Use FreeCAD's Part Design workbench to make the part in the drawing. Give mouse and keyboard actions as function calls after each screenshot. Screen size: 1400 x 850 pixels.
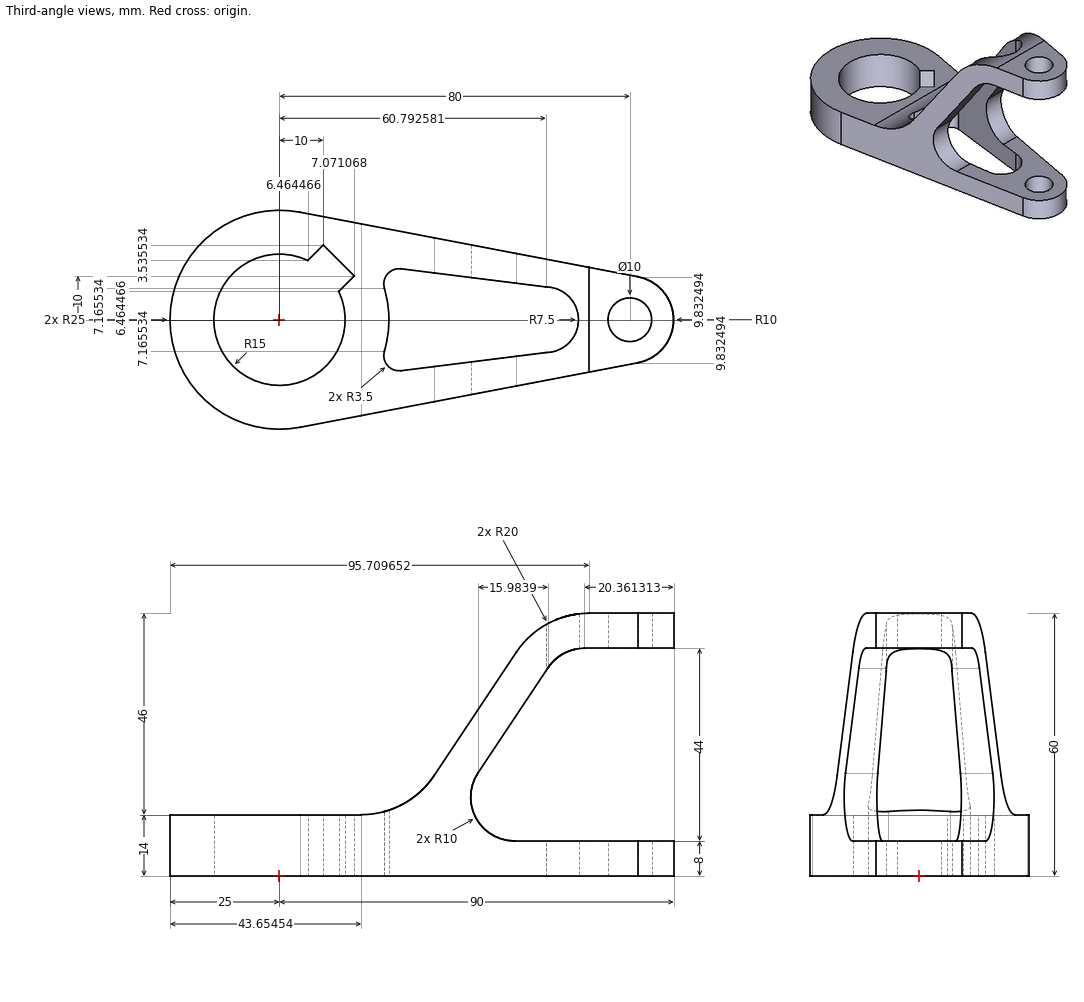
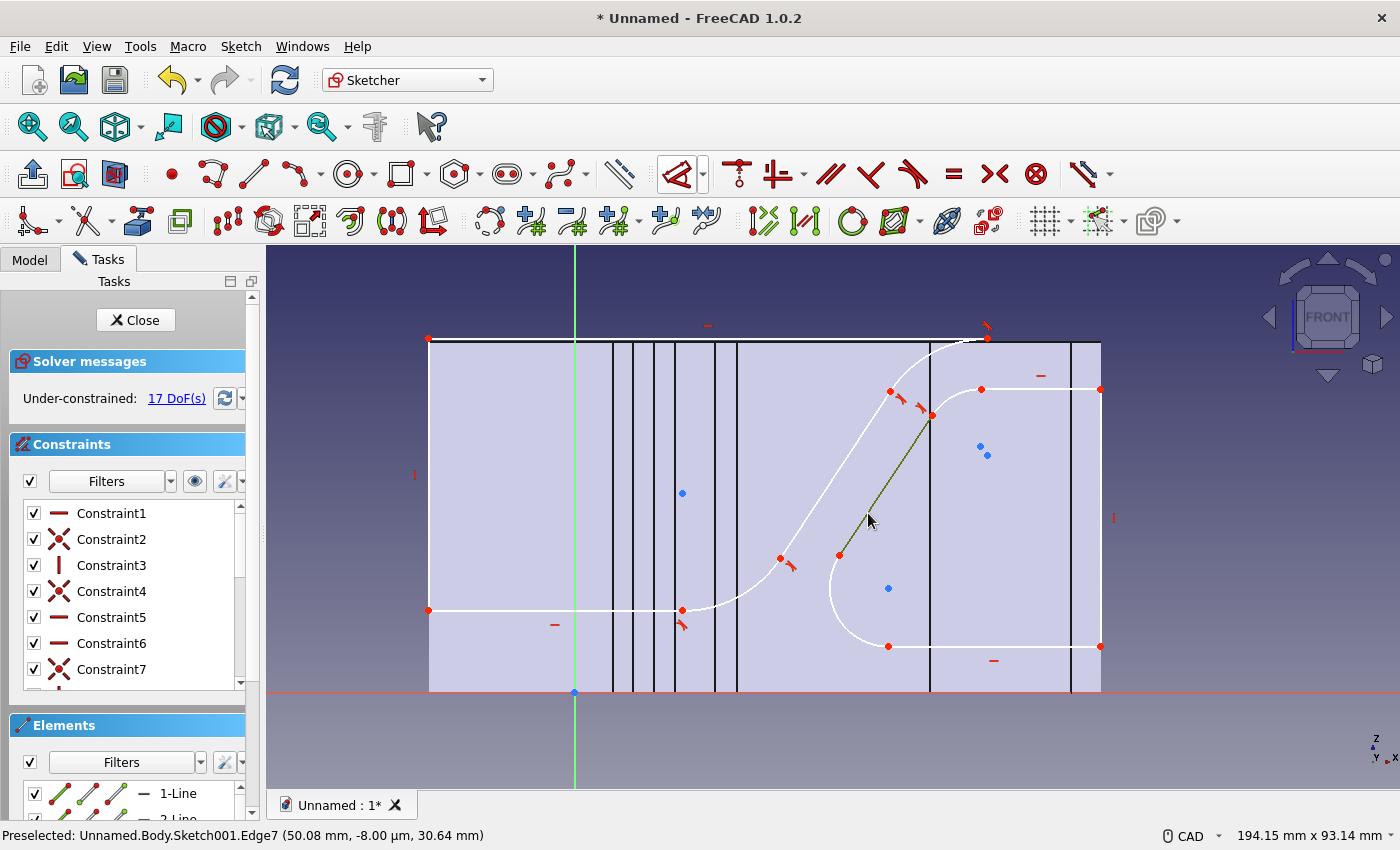
click(830, 592)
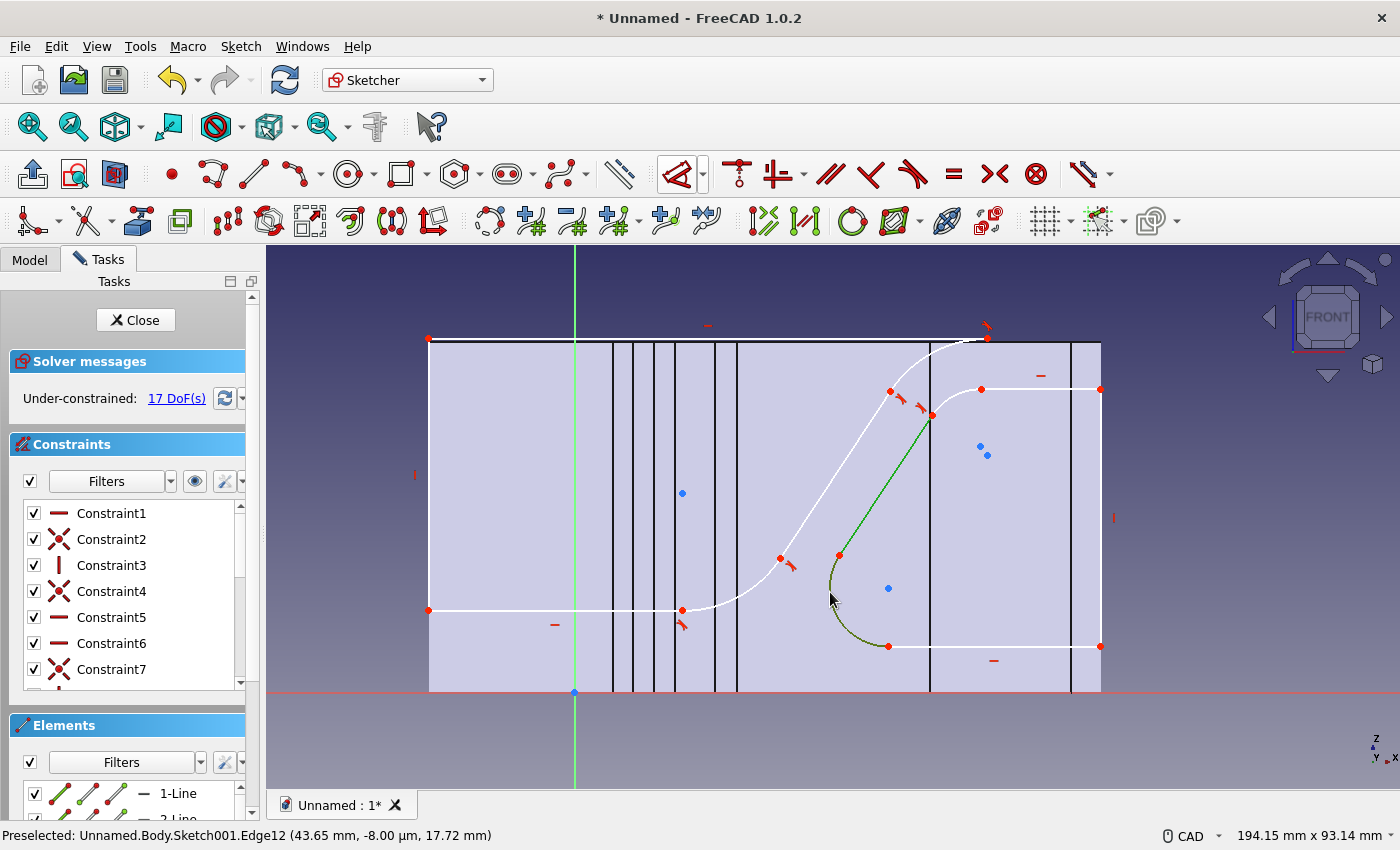
click(913, 174)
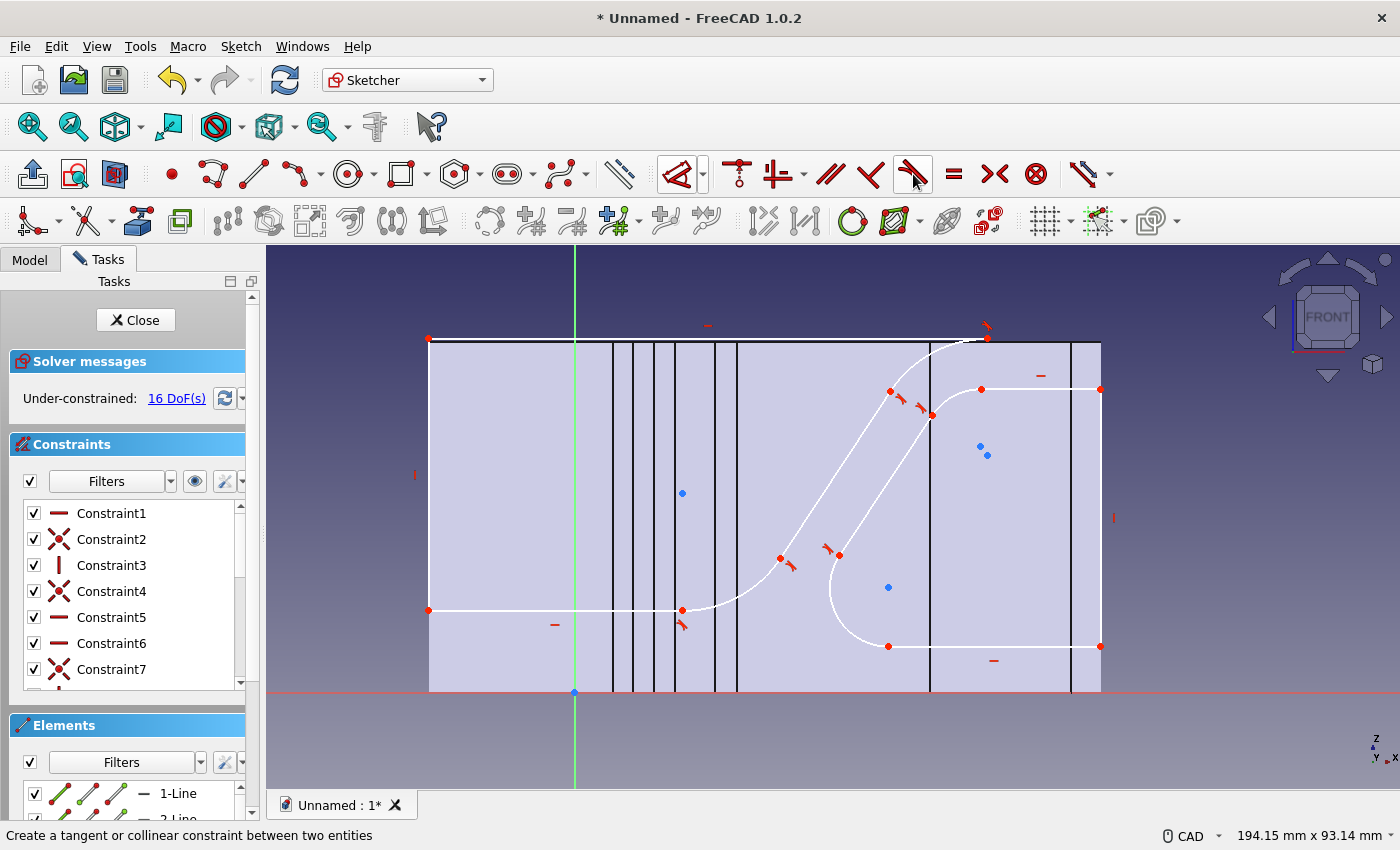
click(1017, 389)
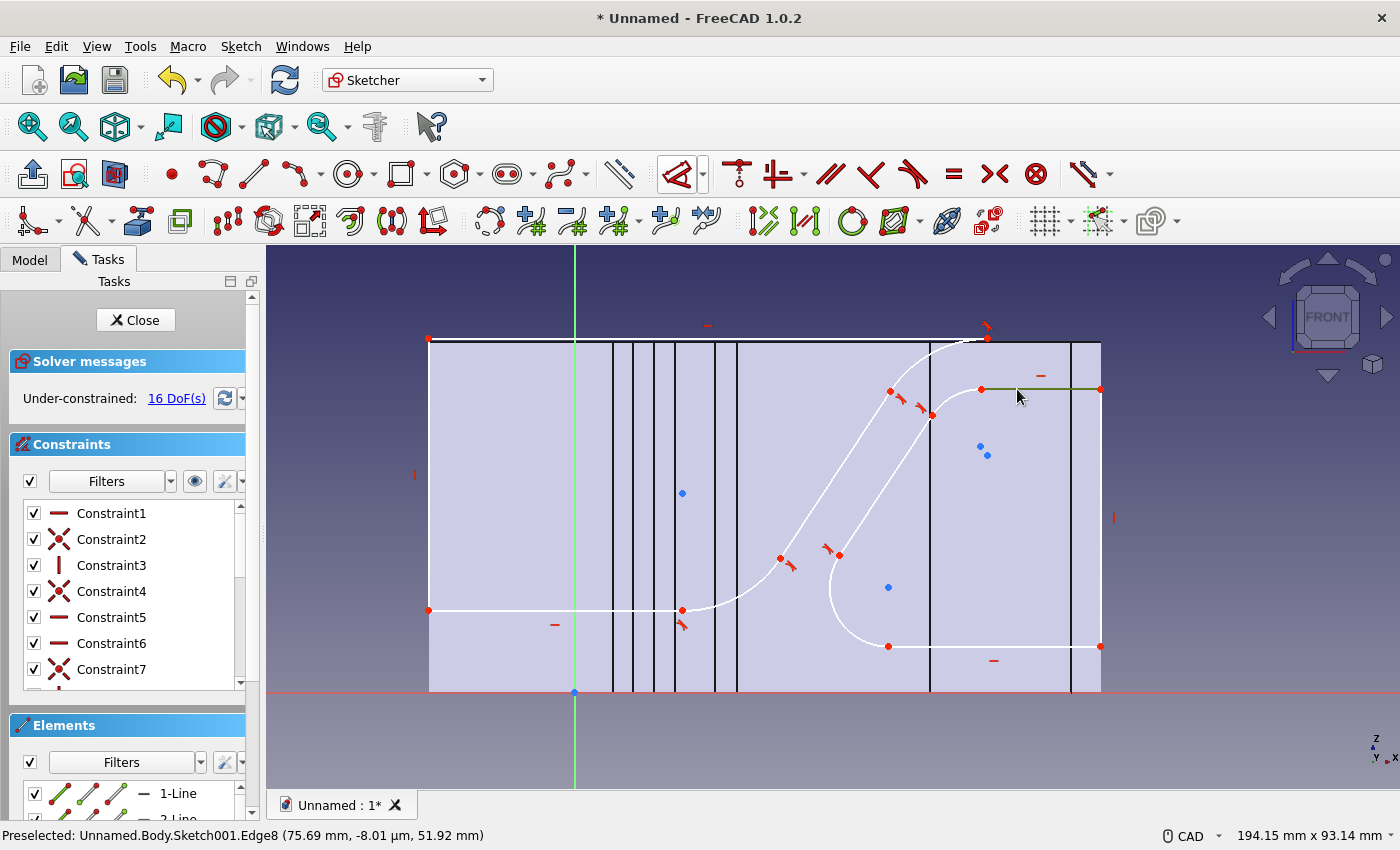
click(965, 392)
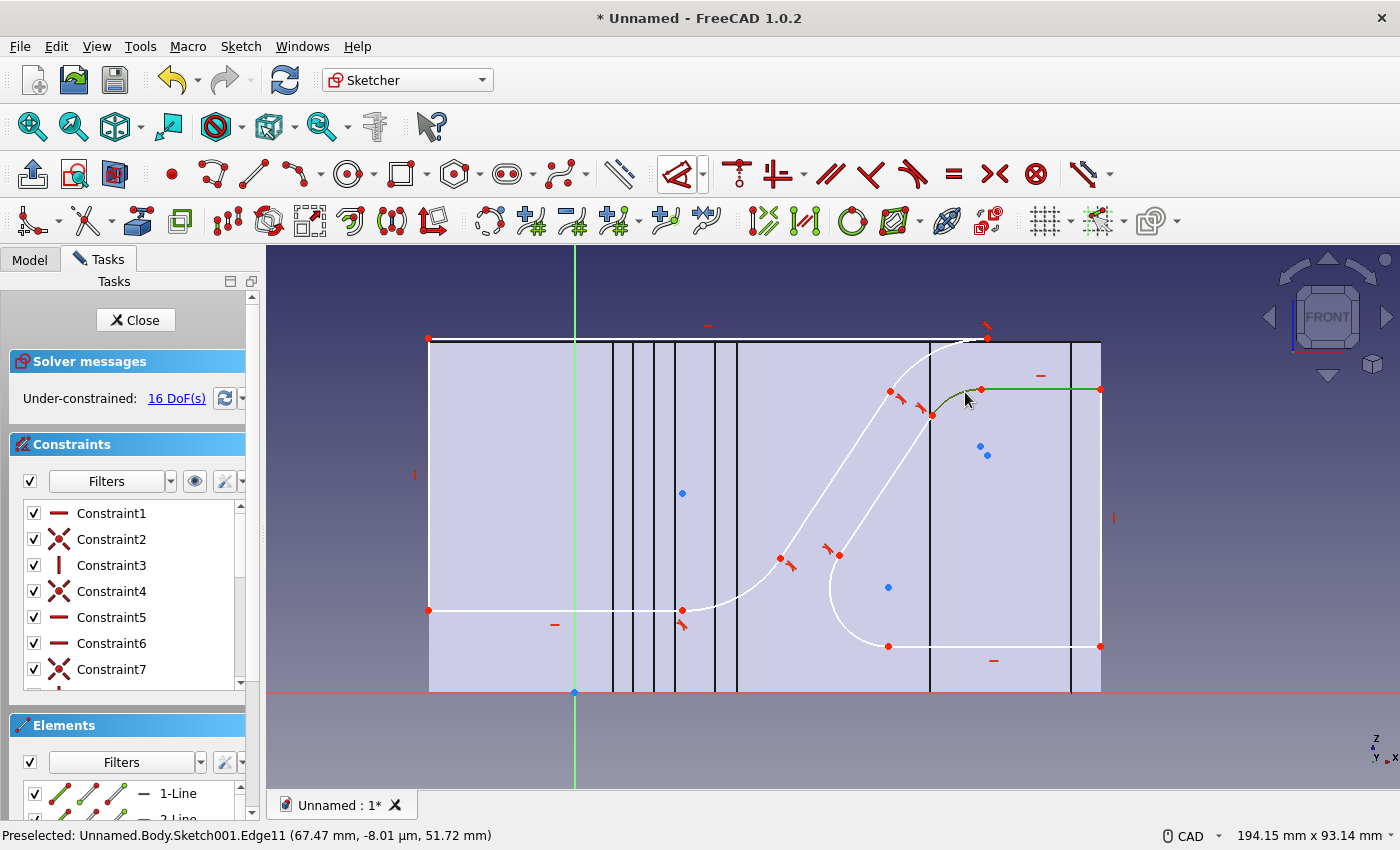
click(913, 174)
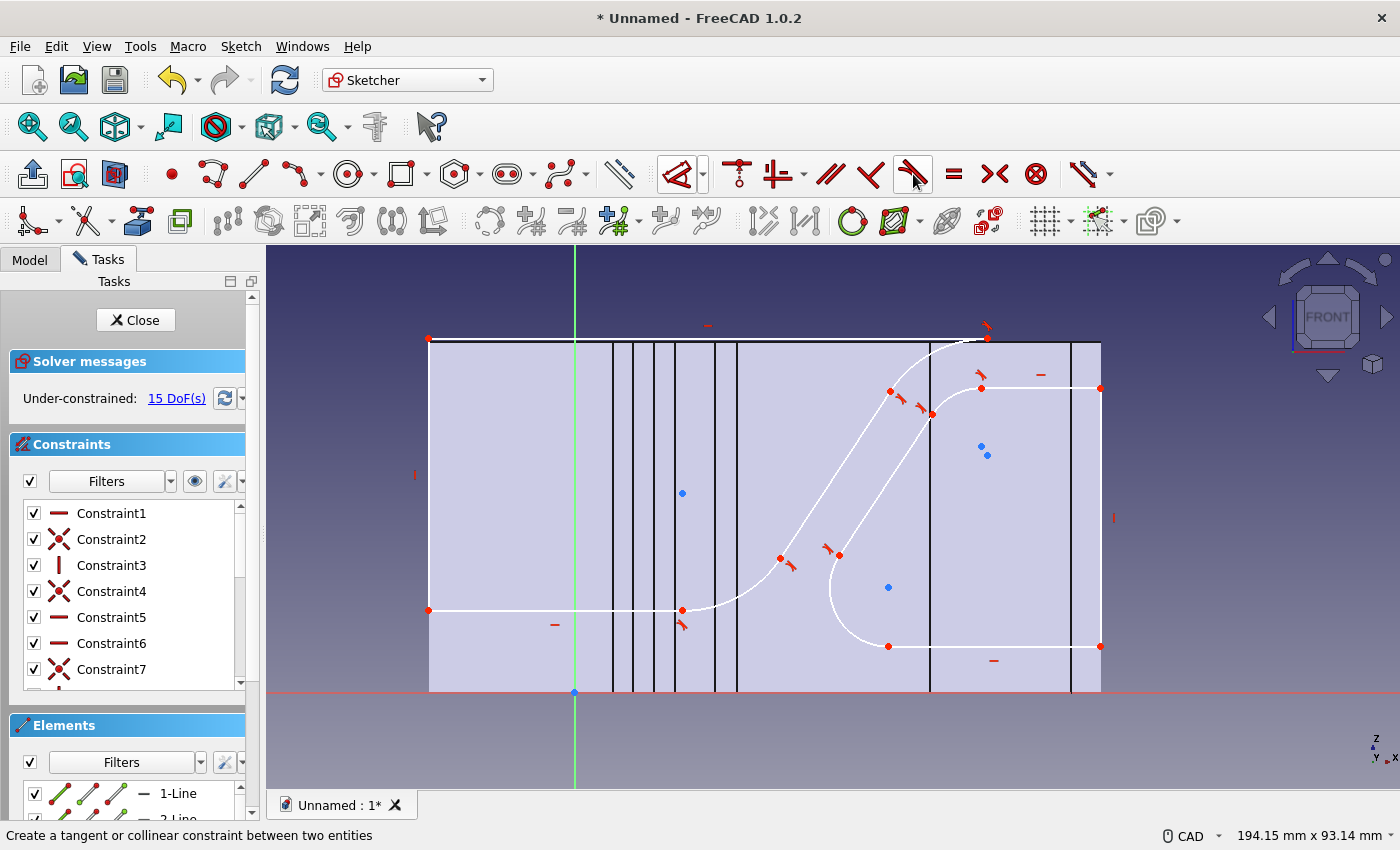
click(1037, 647)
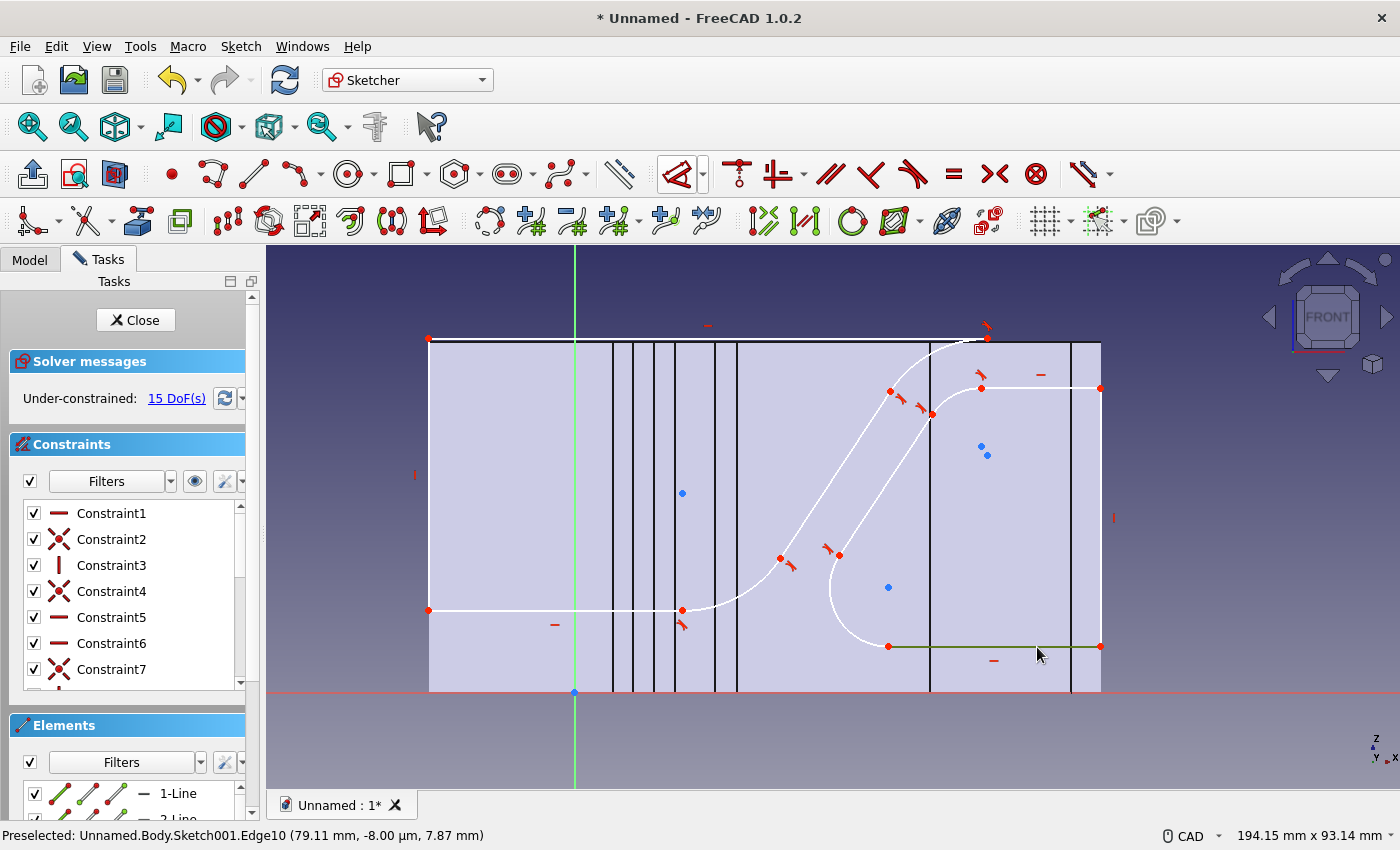
click(830, 592)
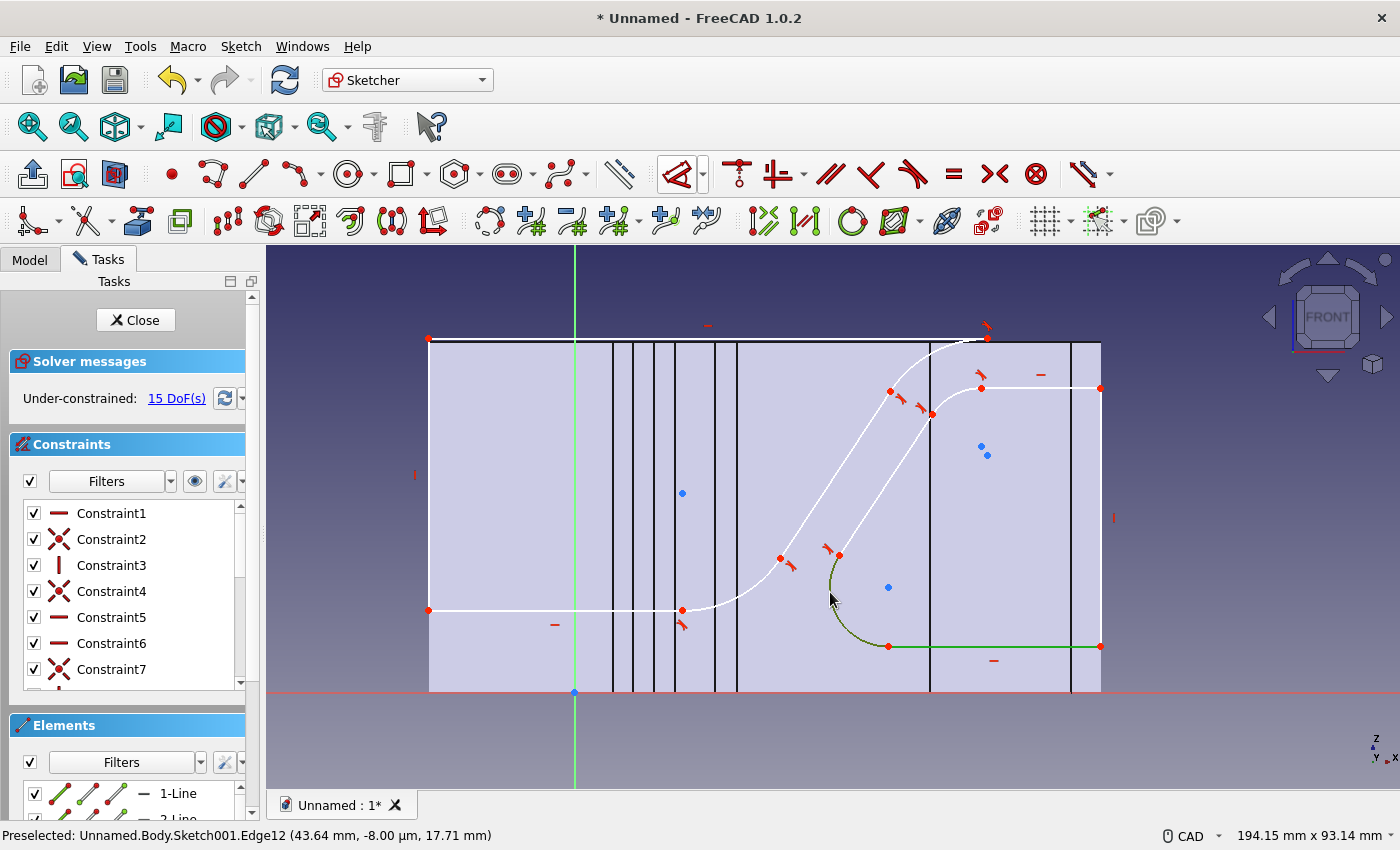
click(913, 174)